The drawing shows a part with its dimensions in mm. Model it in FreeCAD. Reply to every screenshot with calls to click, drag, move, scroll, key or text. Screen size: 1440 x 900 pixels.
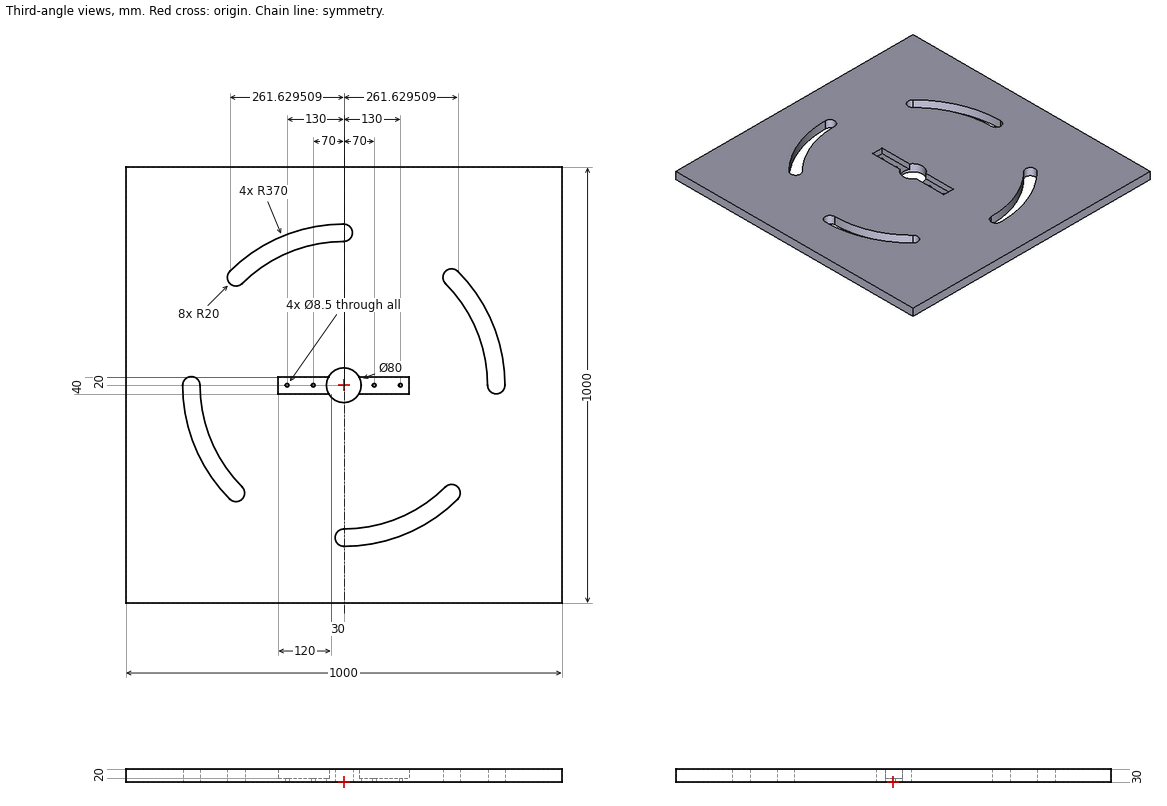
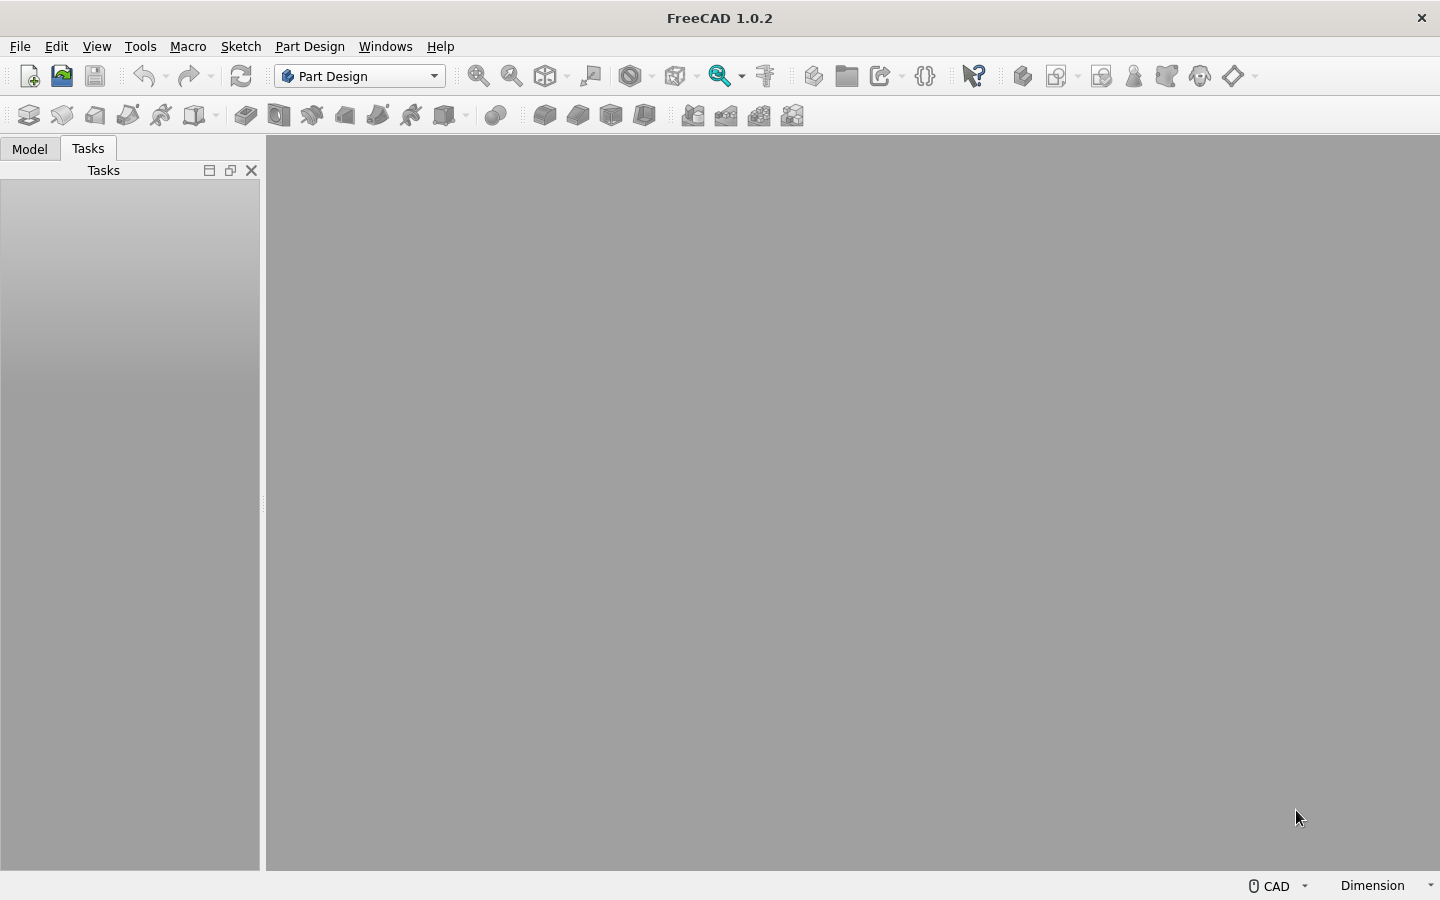
click(29, 76)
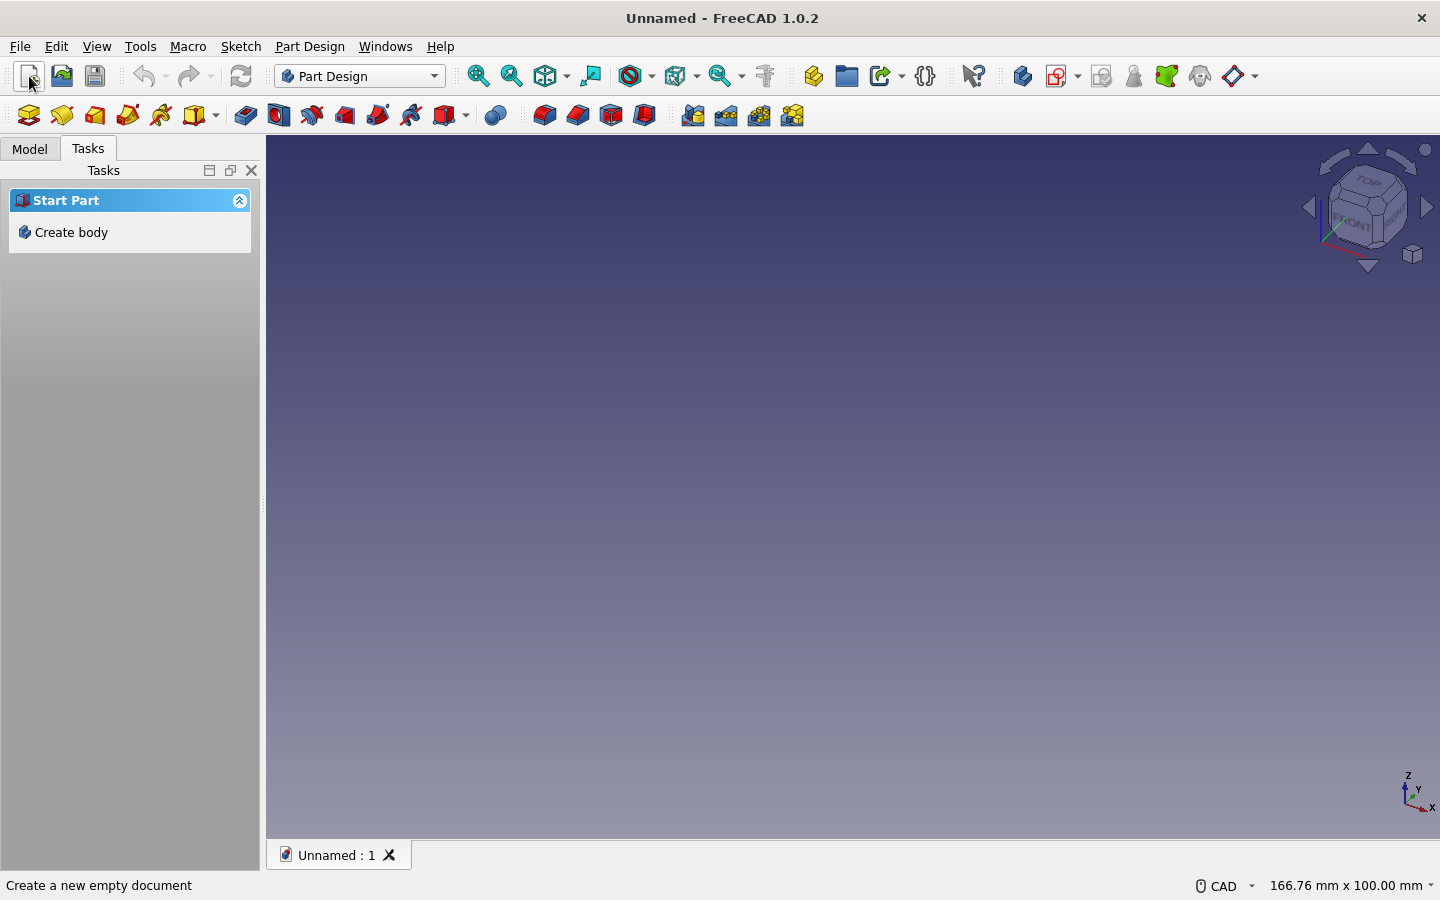
click(1056, 76)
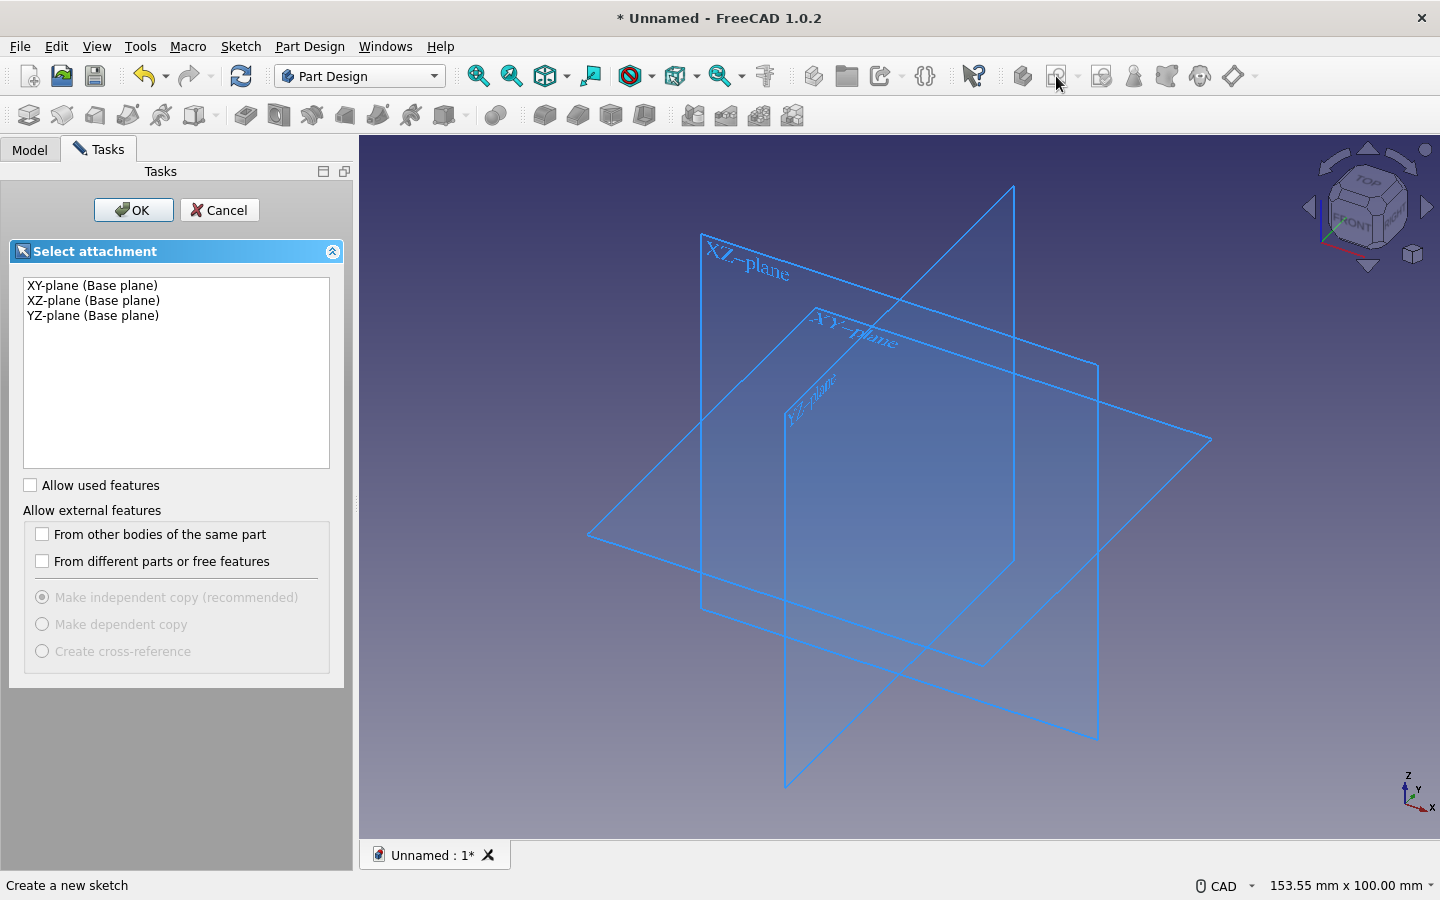
click(84, 286)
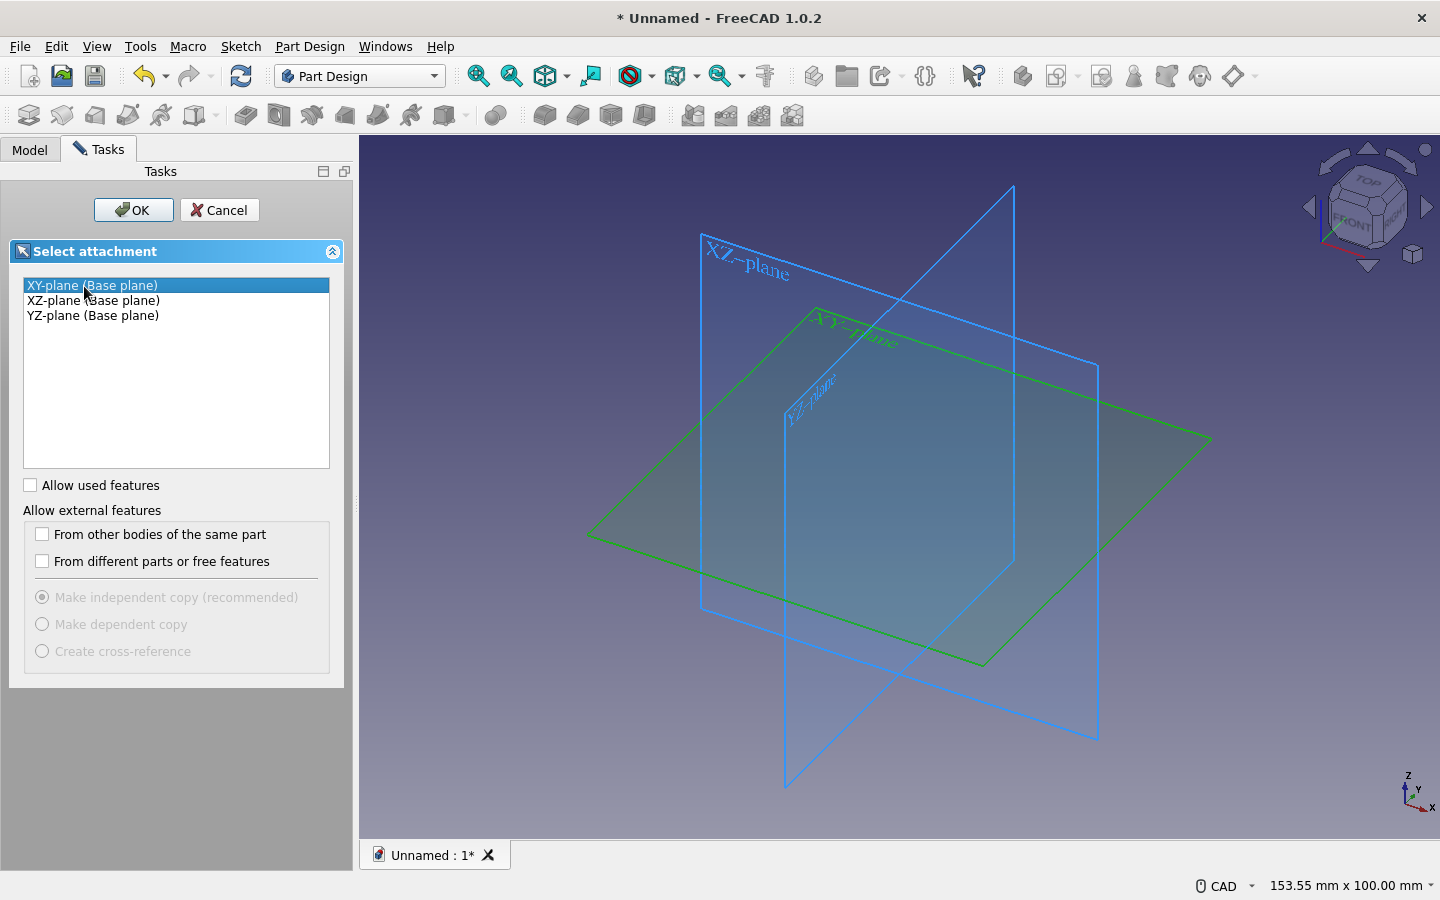
click(134, 210)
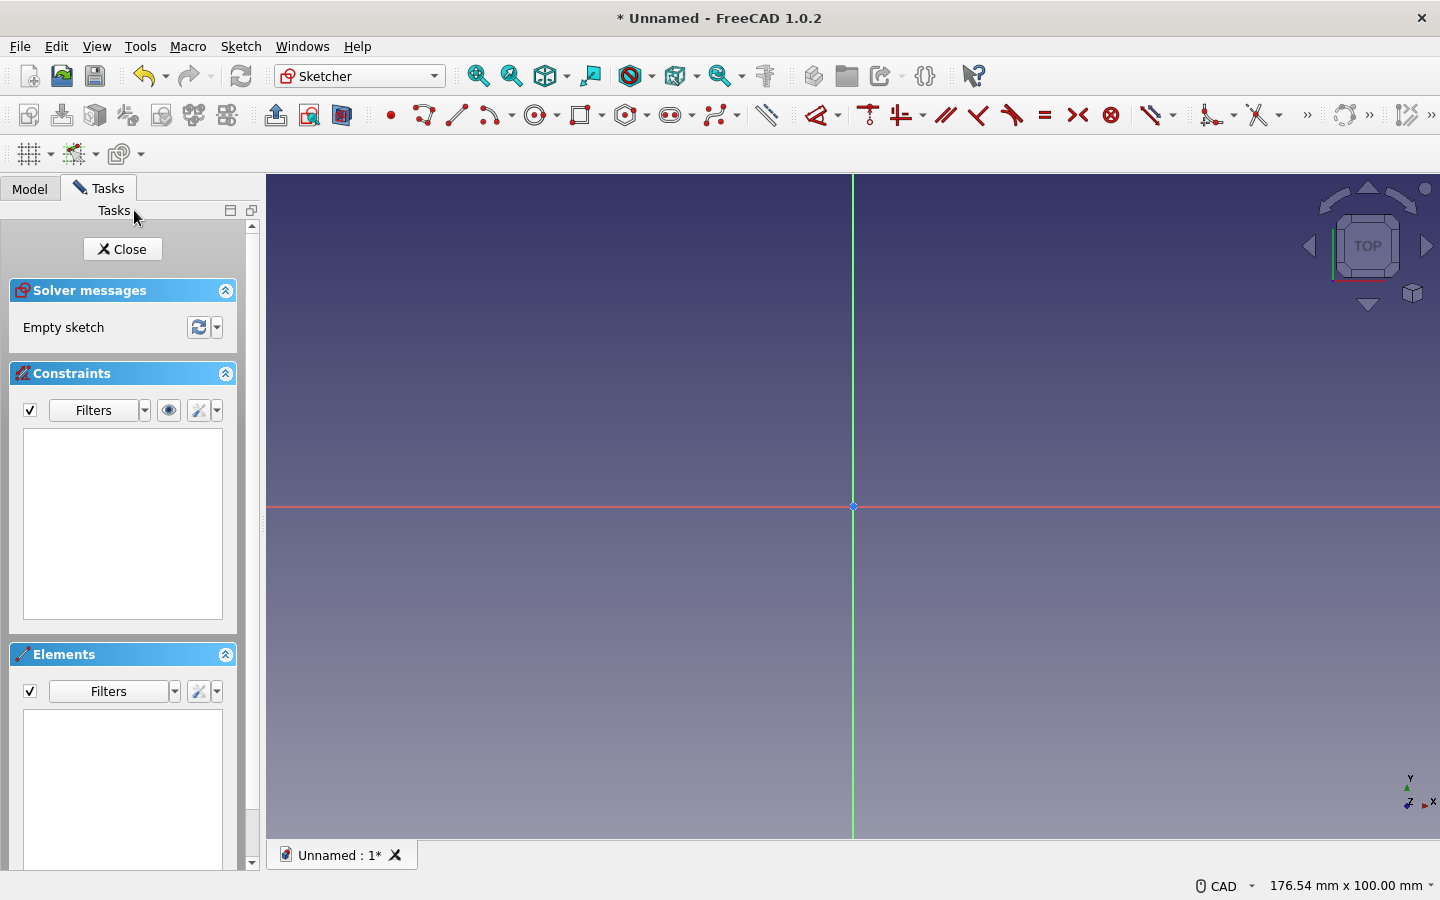
scroll(780, 506, down, 14)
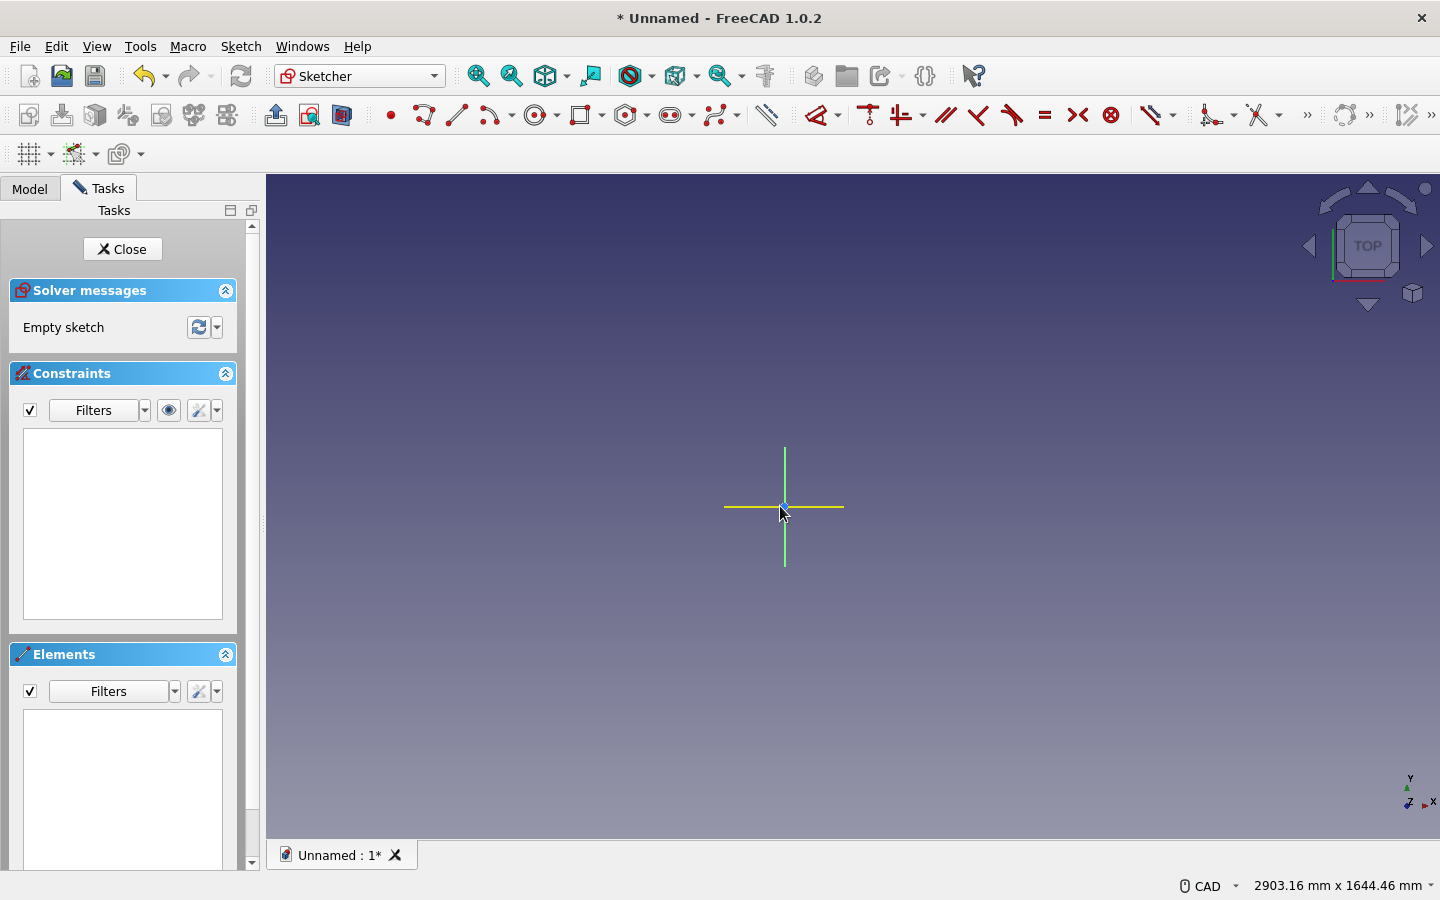
click(602, 116)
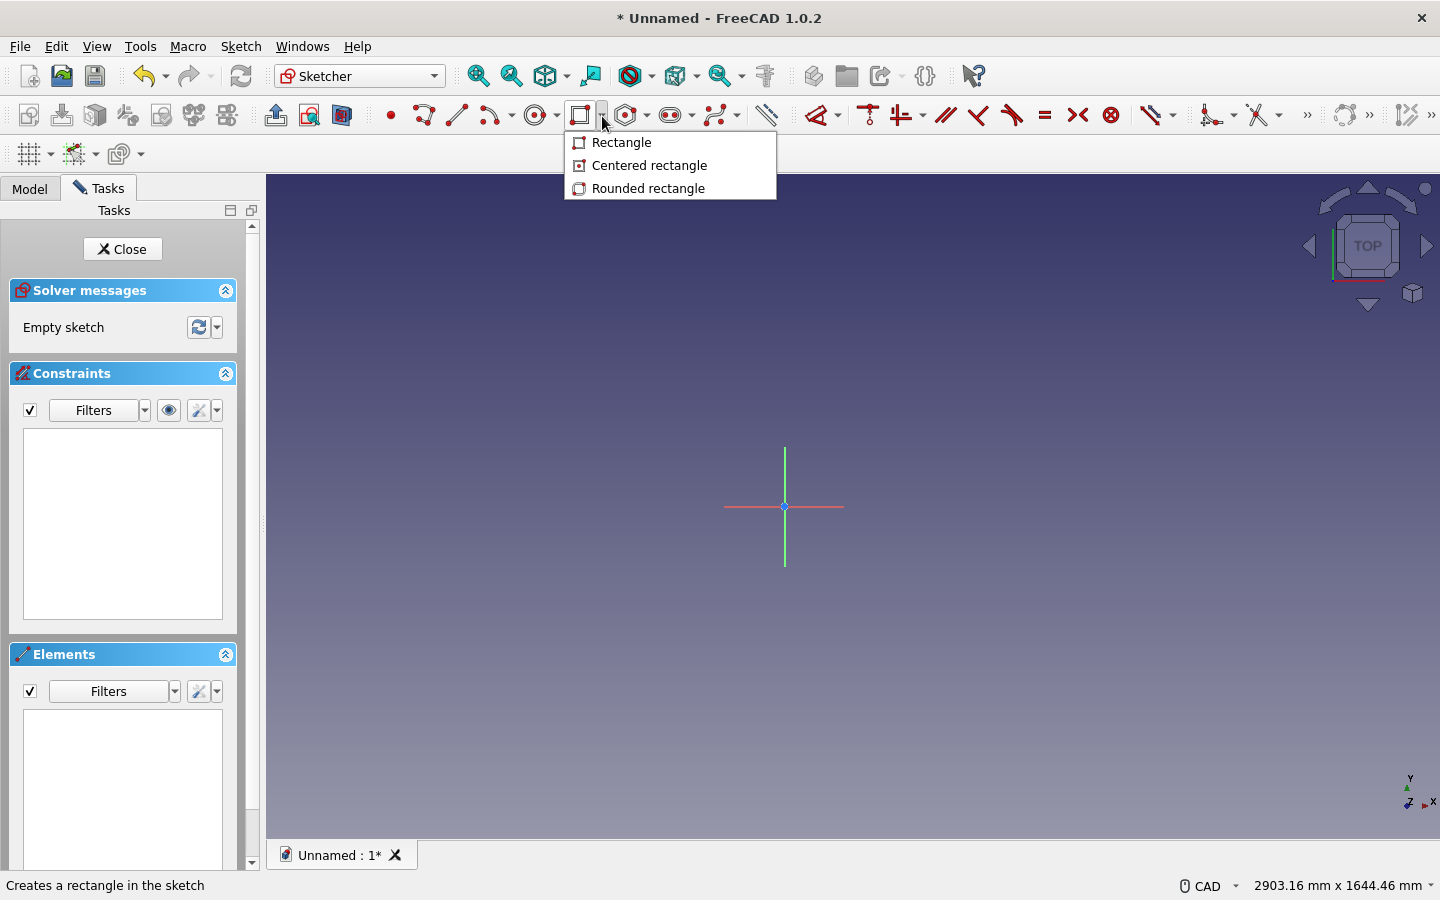
click(670, 166)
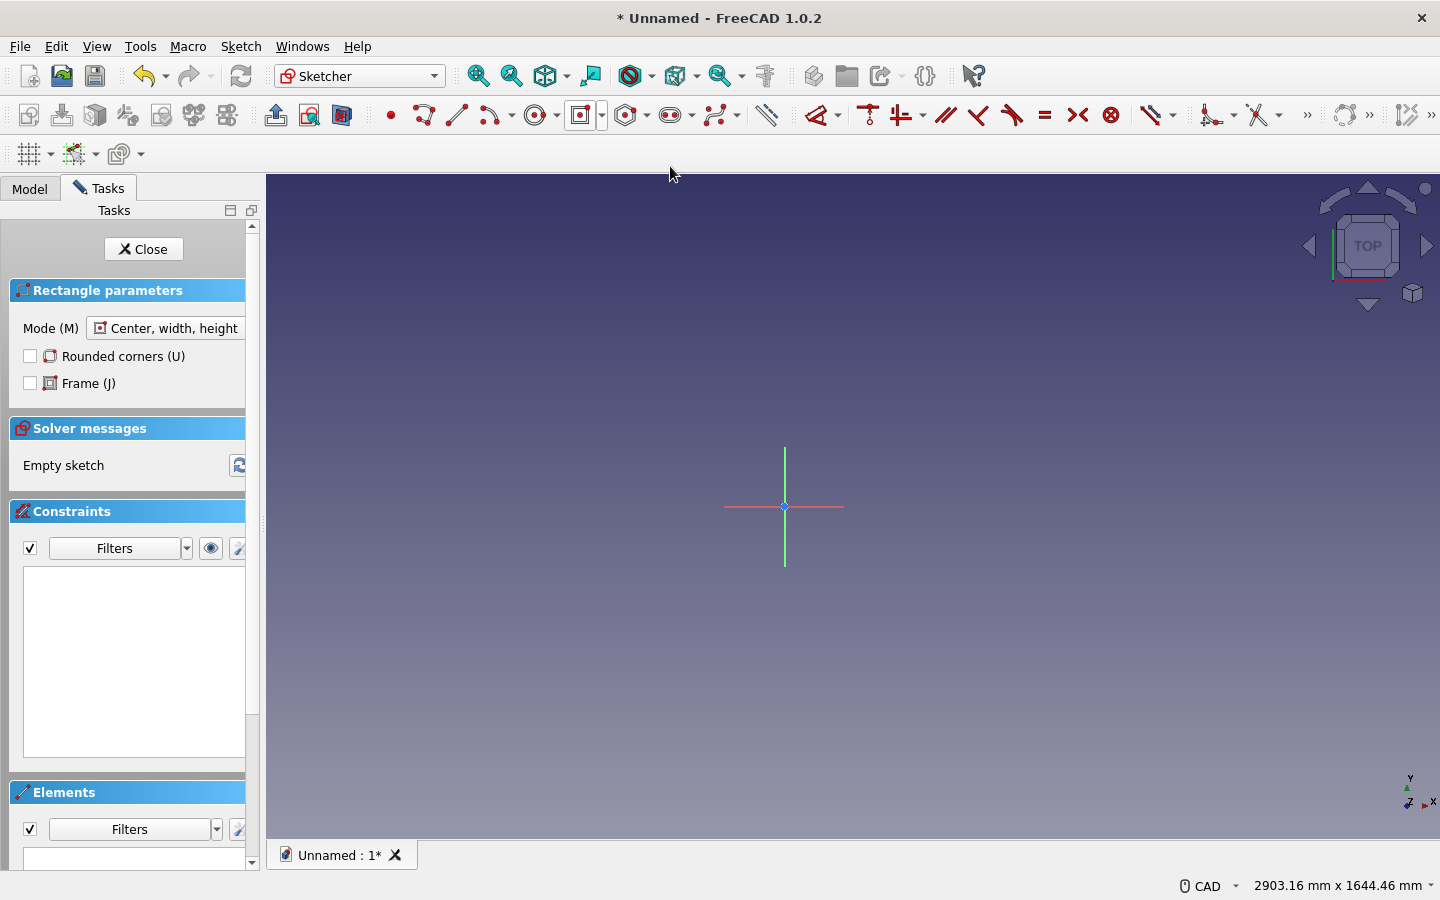
click(785, 506)
click(987, 304)
key(Escape)